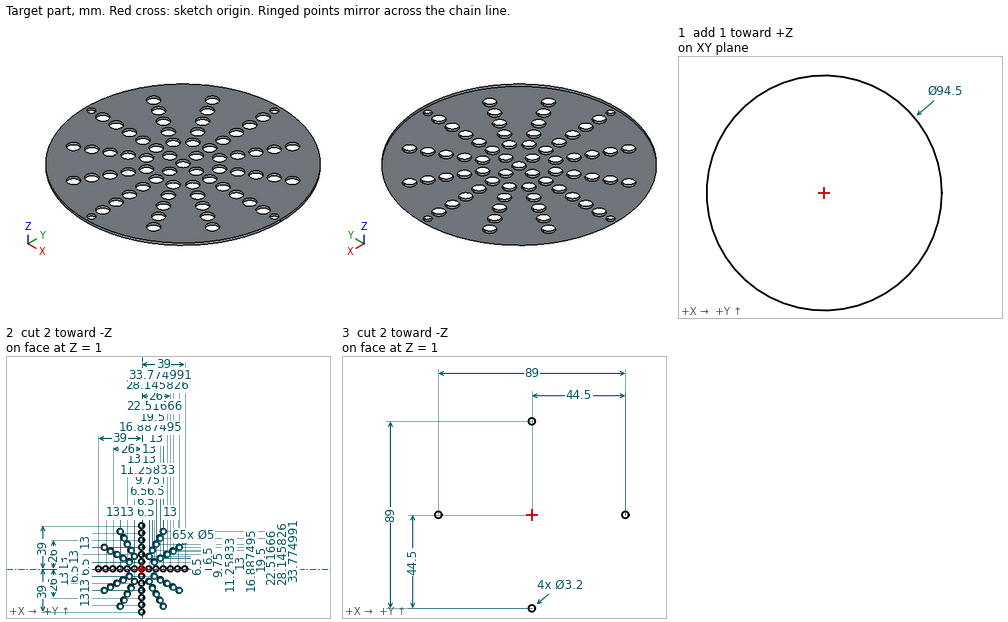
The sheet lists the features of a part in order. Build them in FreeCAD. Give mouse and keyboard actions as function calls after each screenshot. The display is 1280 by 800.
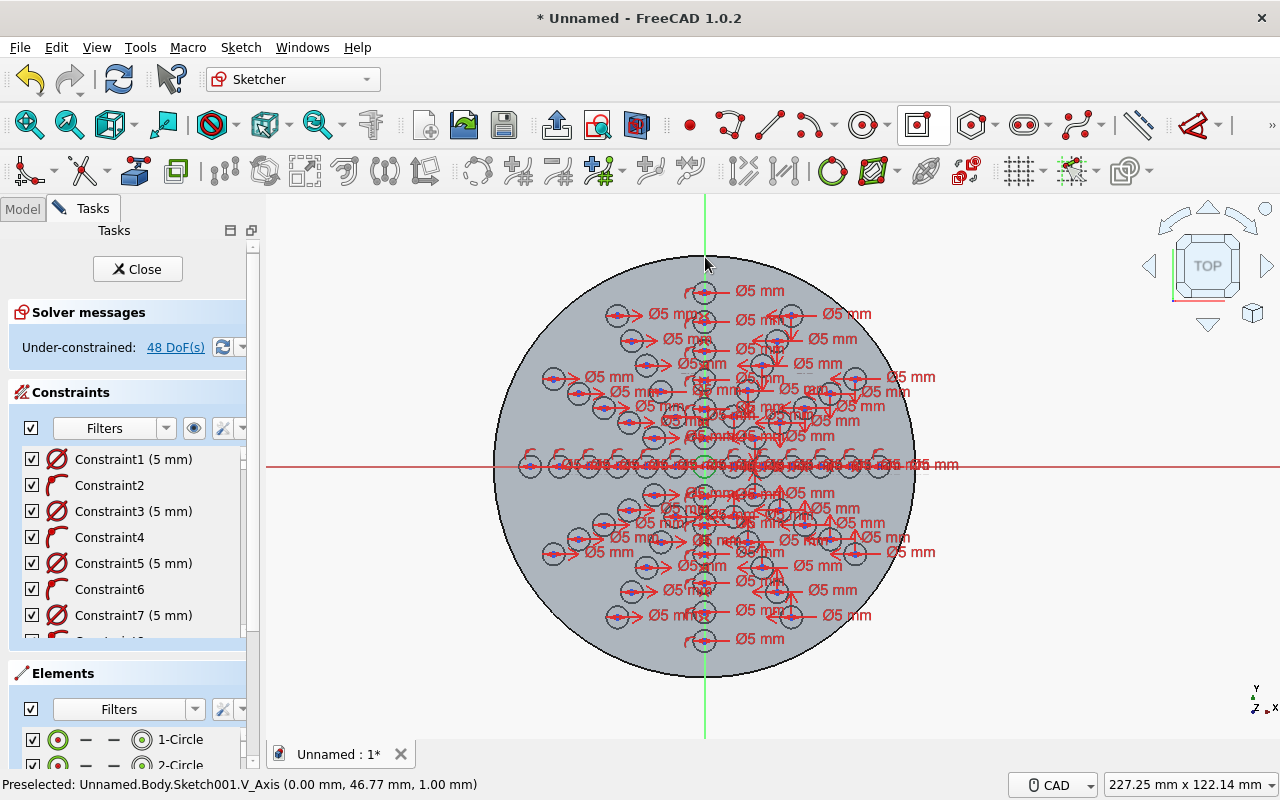
click(748, 391)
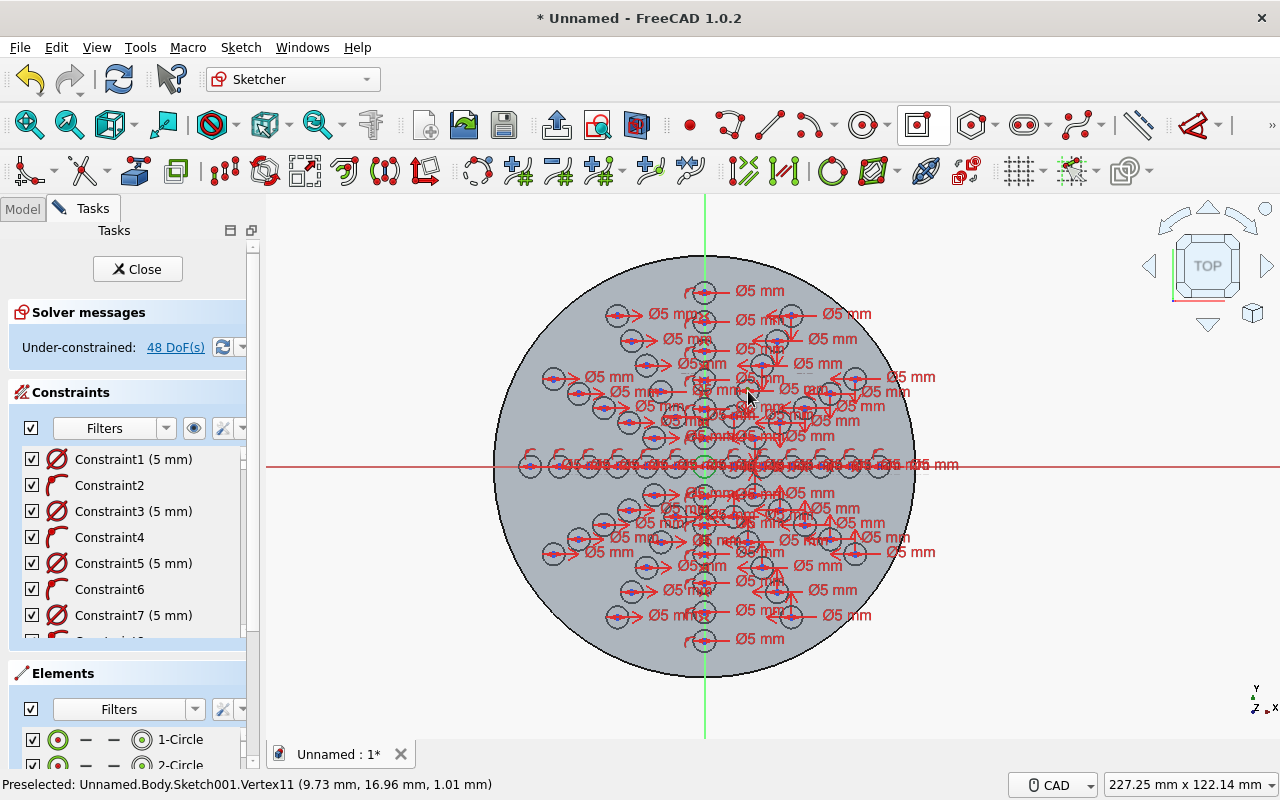
click(661, 392)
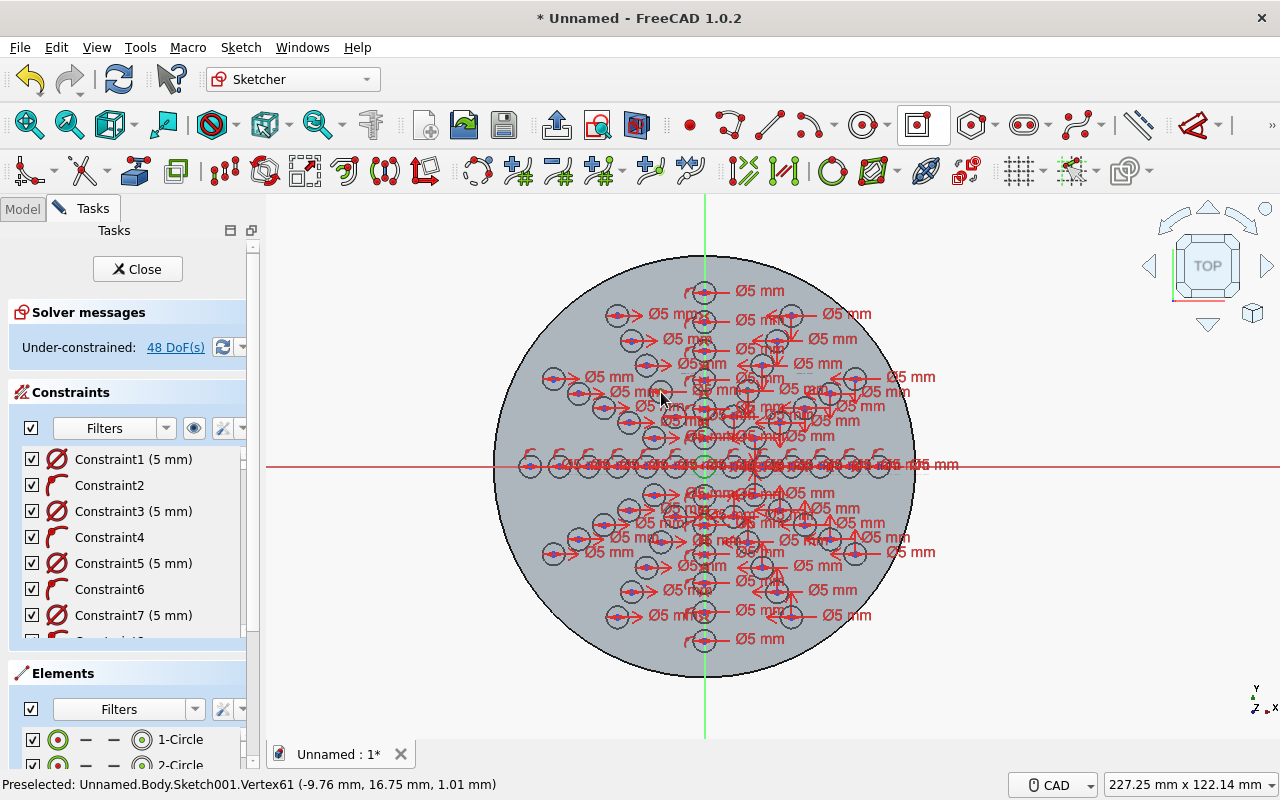
click(705, 257)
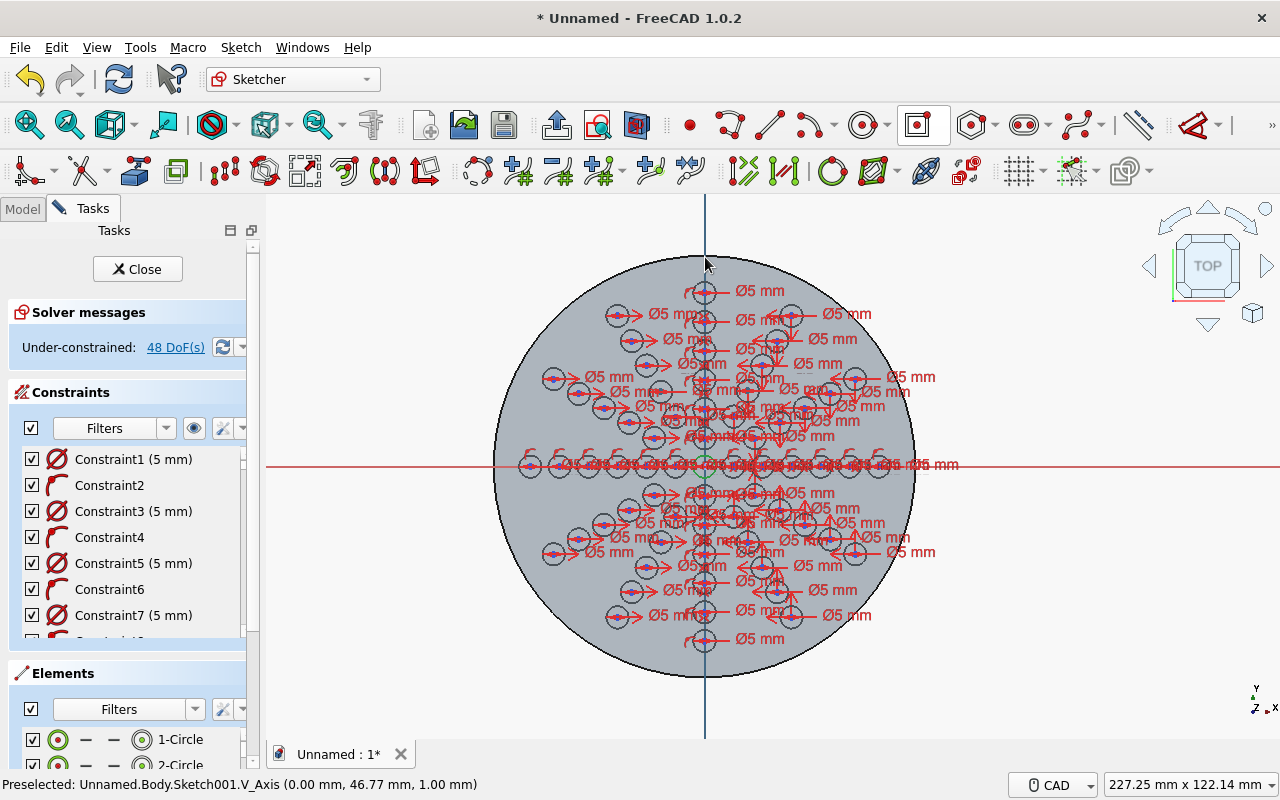
key(s)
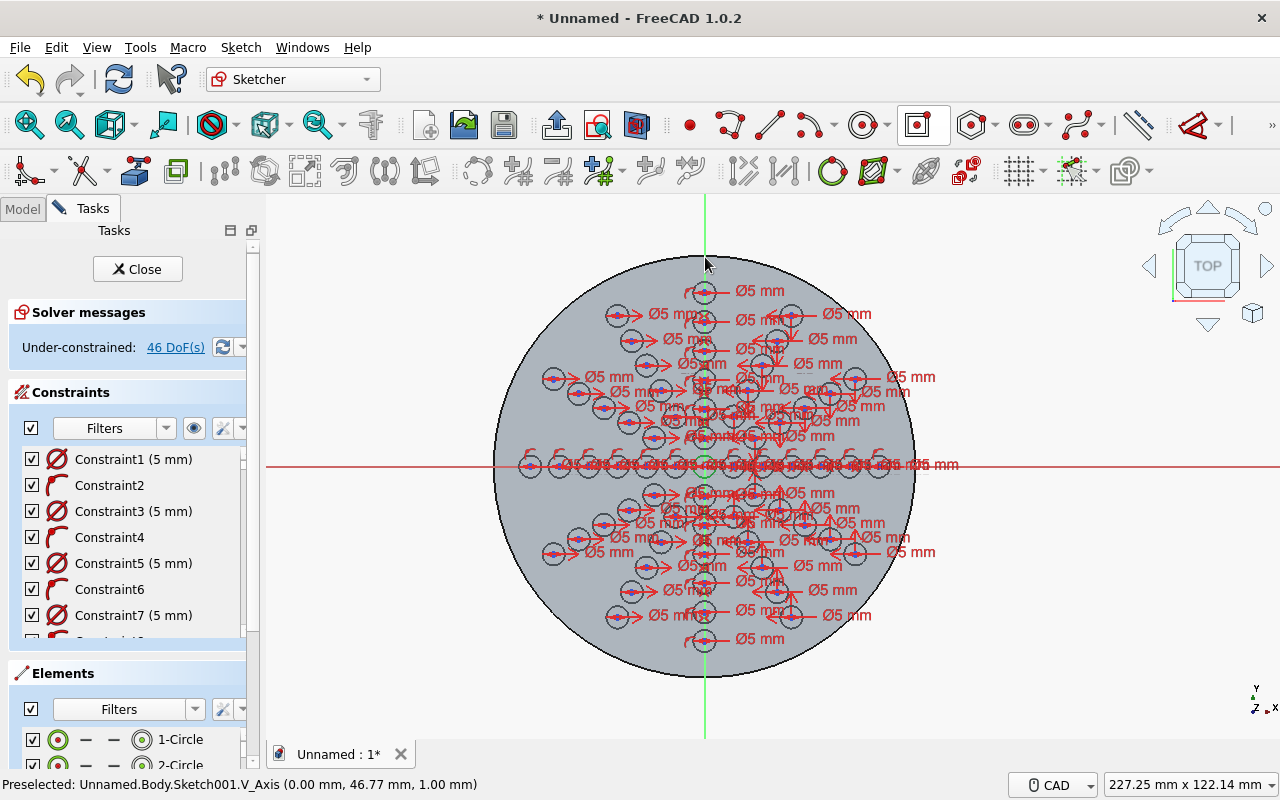
click(734, 417)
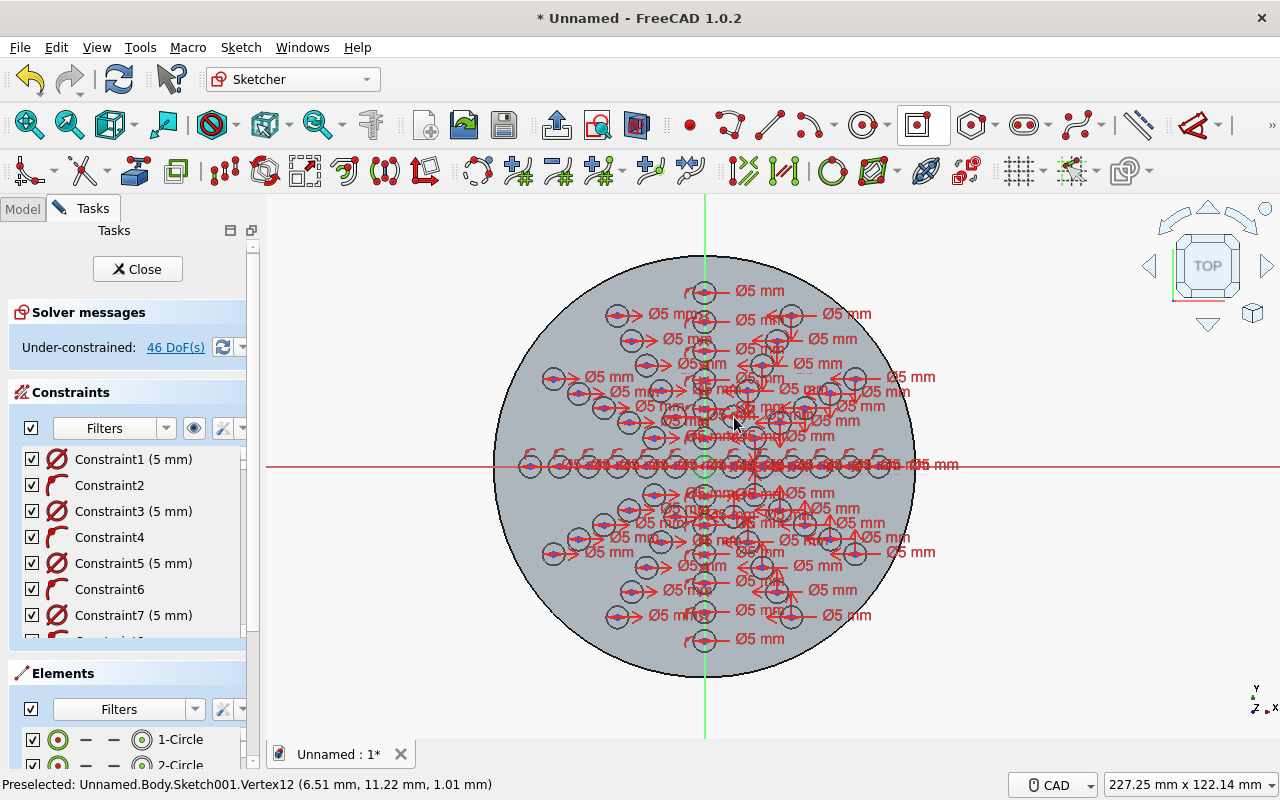
click(675, 417)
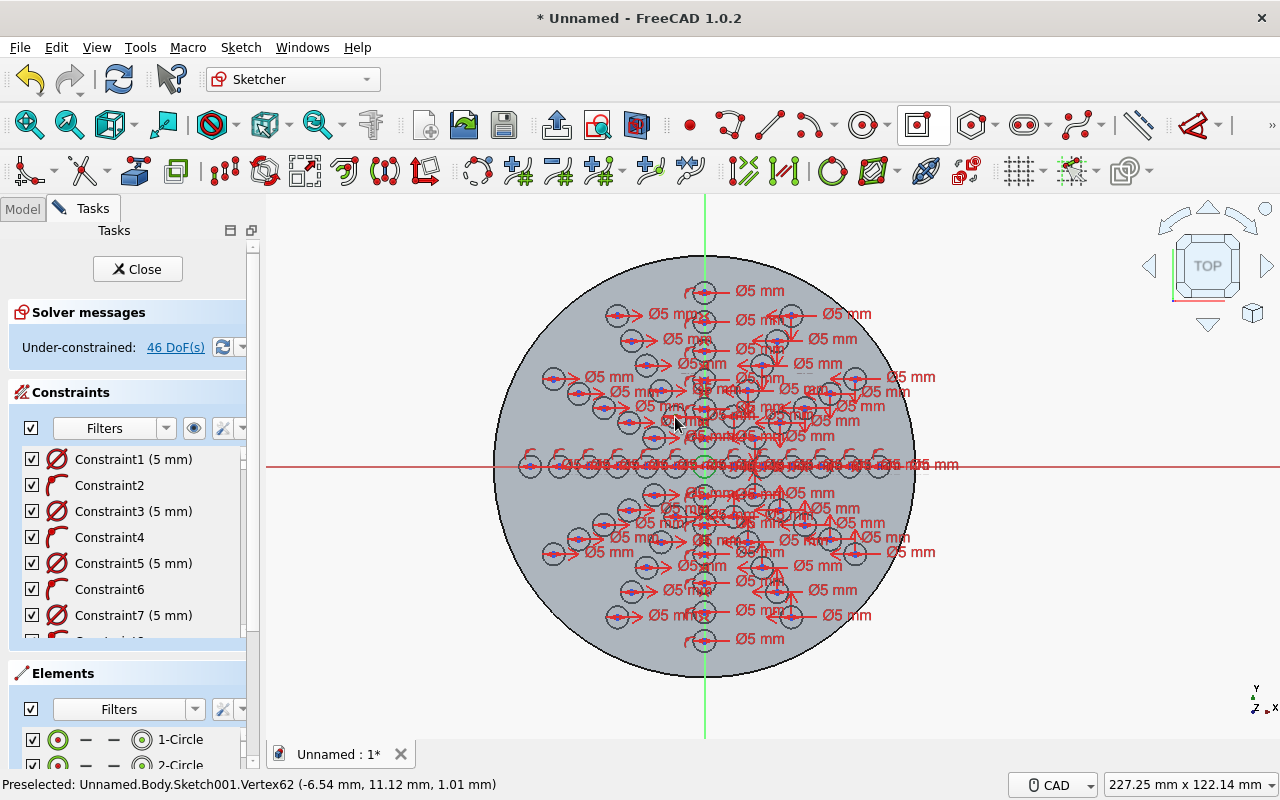
click(705, 257)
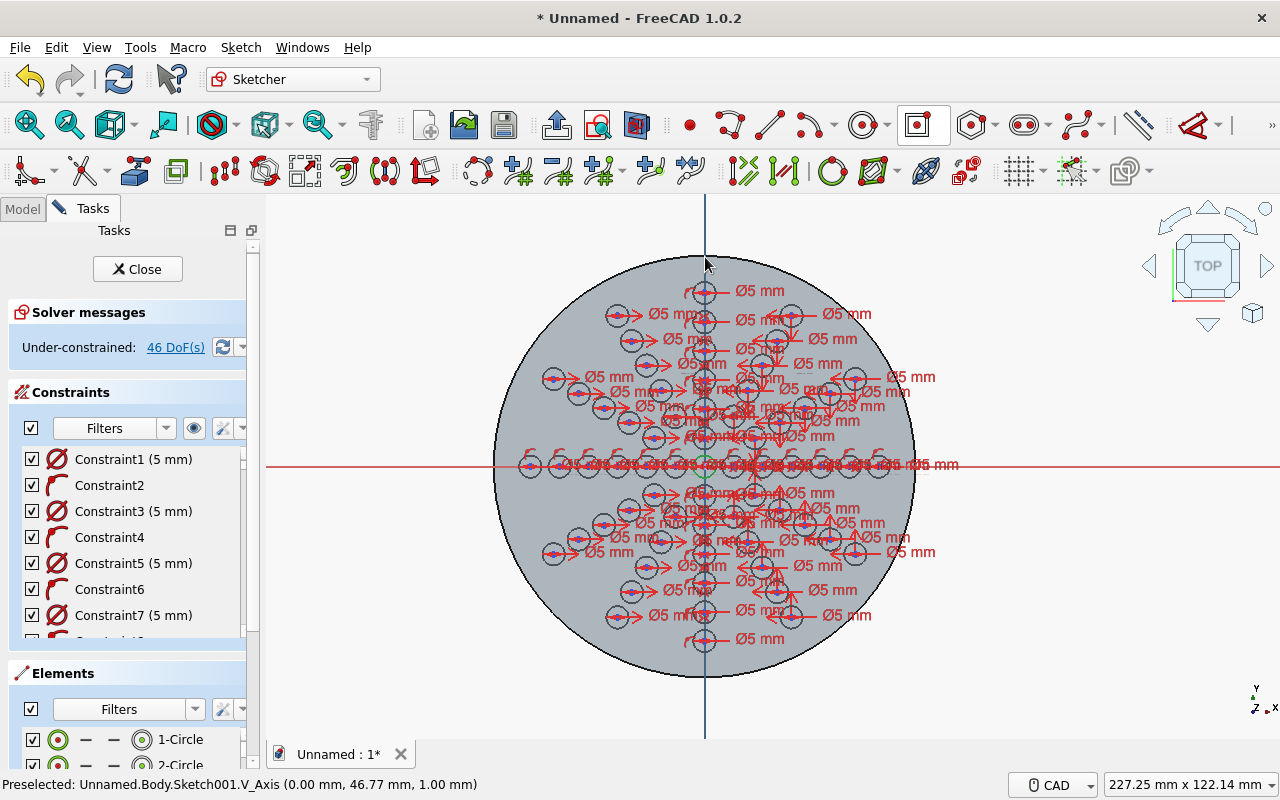
key(s)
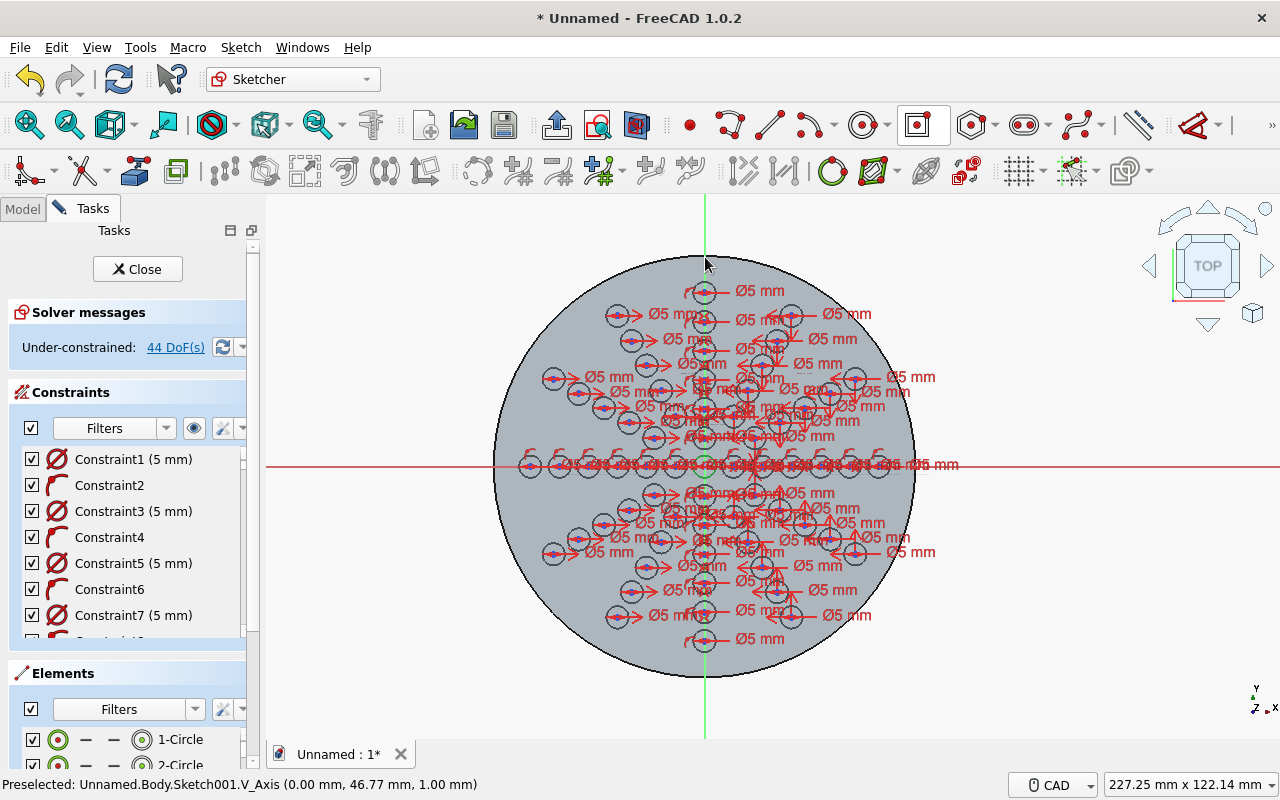
click(1194, 126)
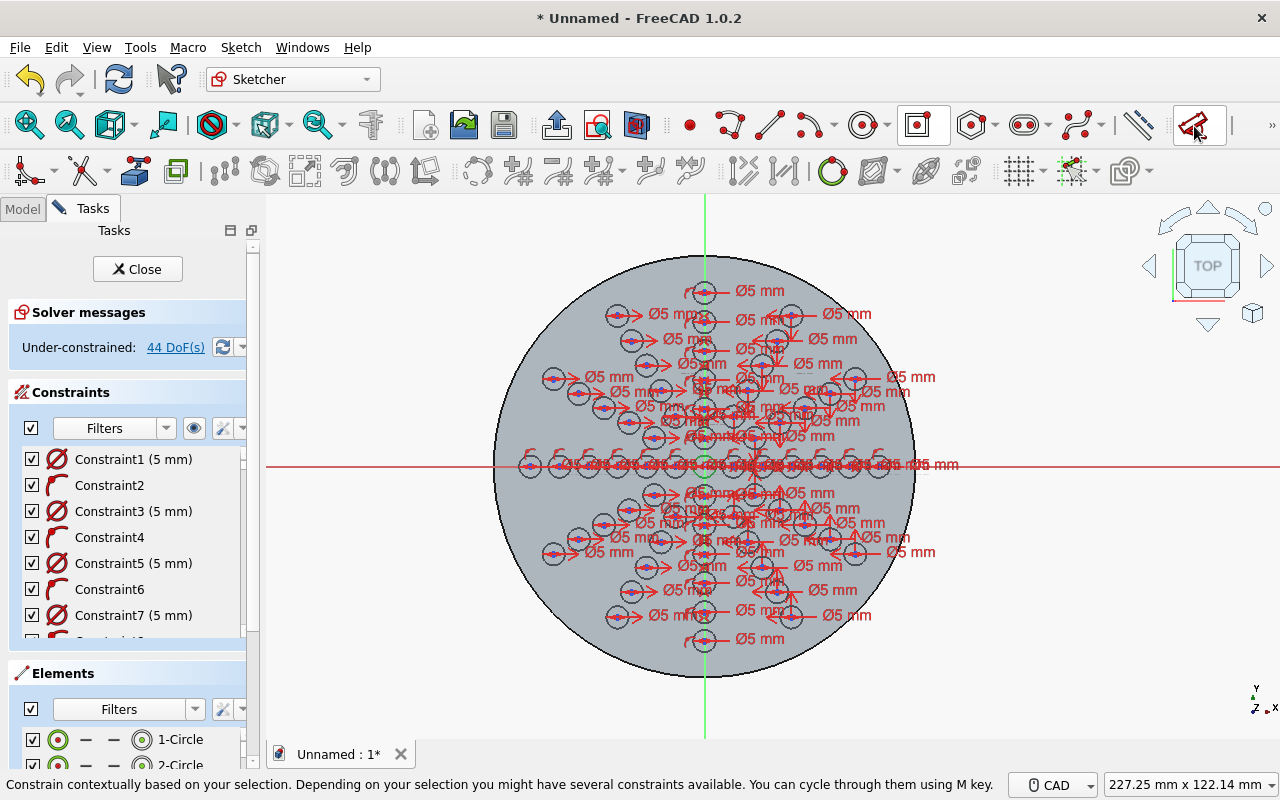
click(705, 409)
click(811, 438)